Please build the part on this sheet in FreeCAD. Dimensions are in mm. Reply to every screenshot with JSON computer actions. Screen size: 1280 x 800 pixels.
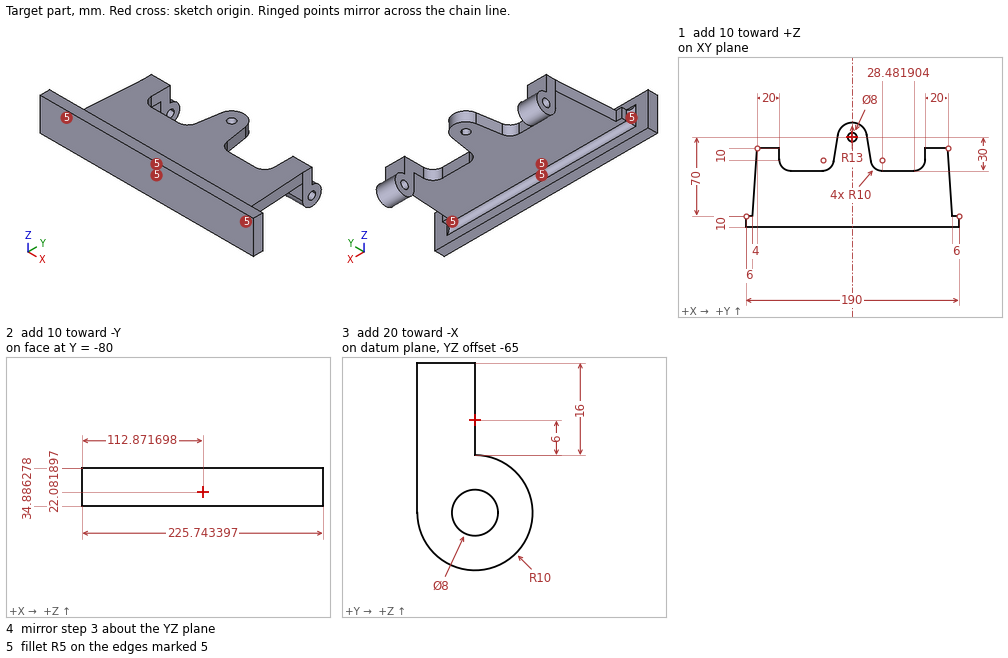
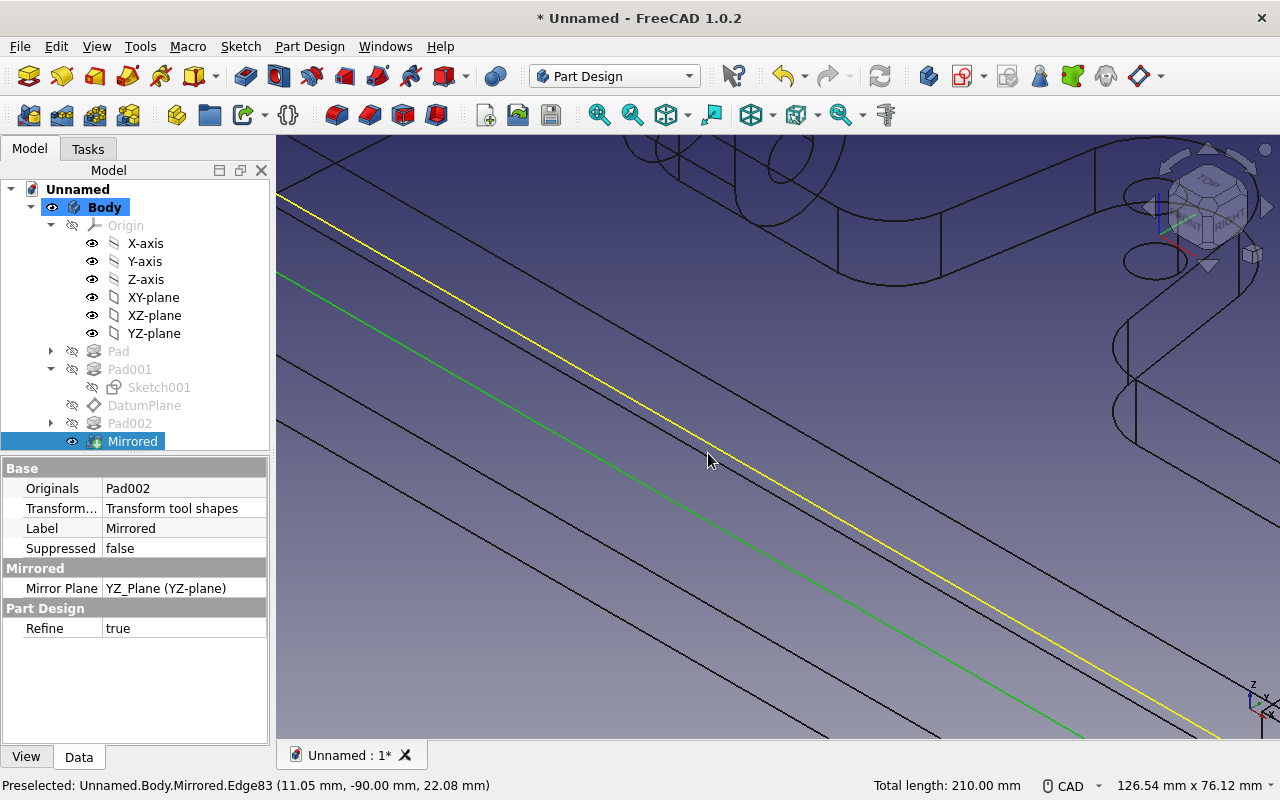
{"action": "left_click", "coordinate": [707, 455], "text": "ctrl"}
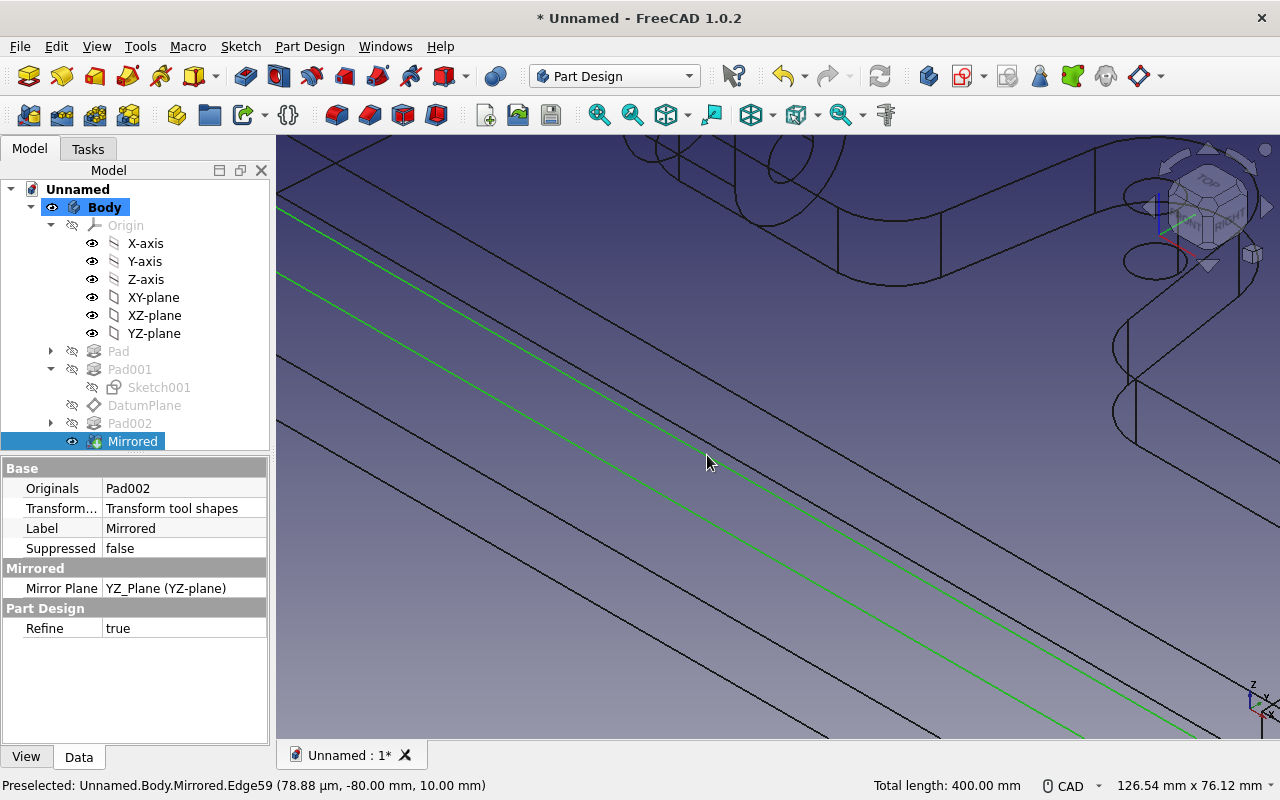
{"action": "key", "text": "v 1"}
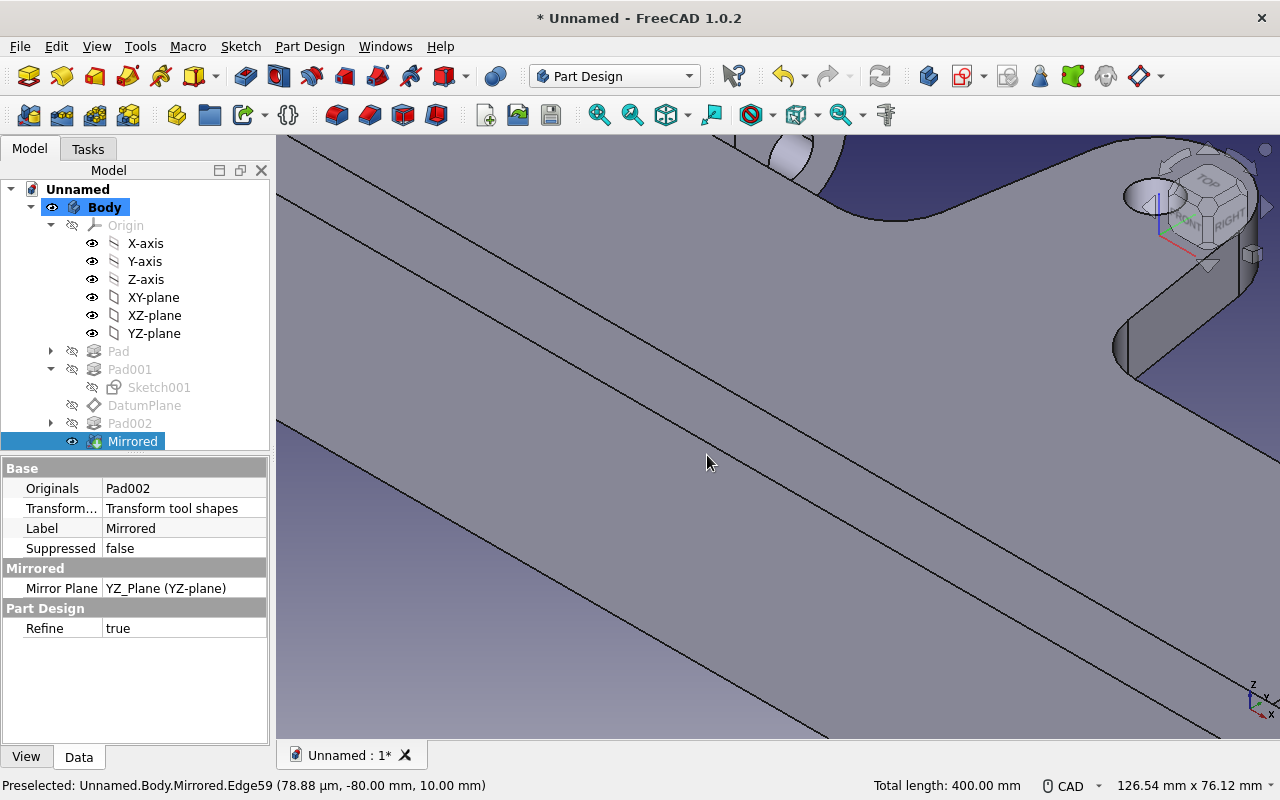
{"action": "left_click", "coordinate": [337, 116]}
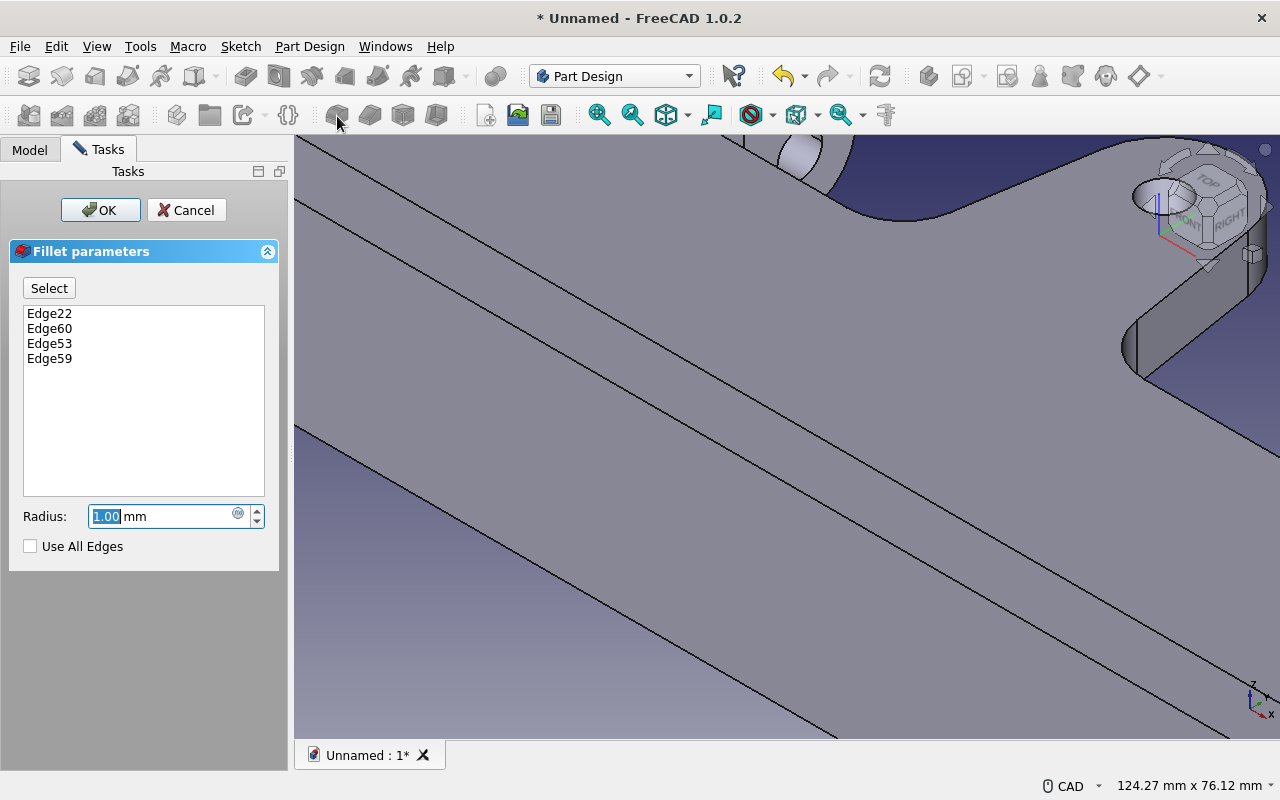
{"action": "type", "text": "5"}
{"action": "key", "text": "Tab"}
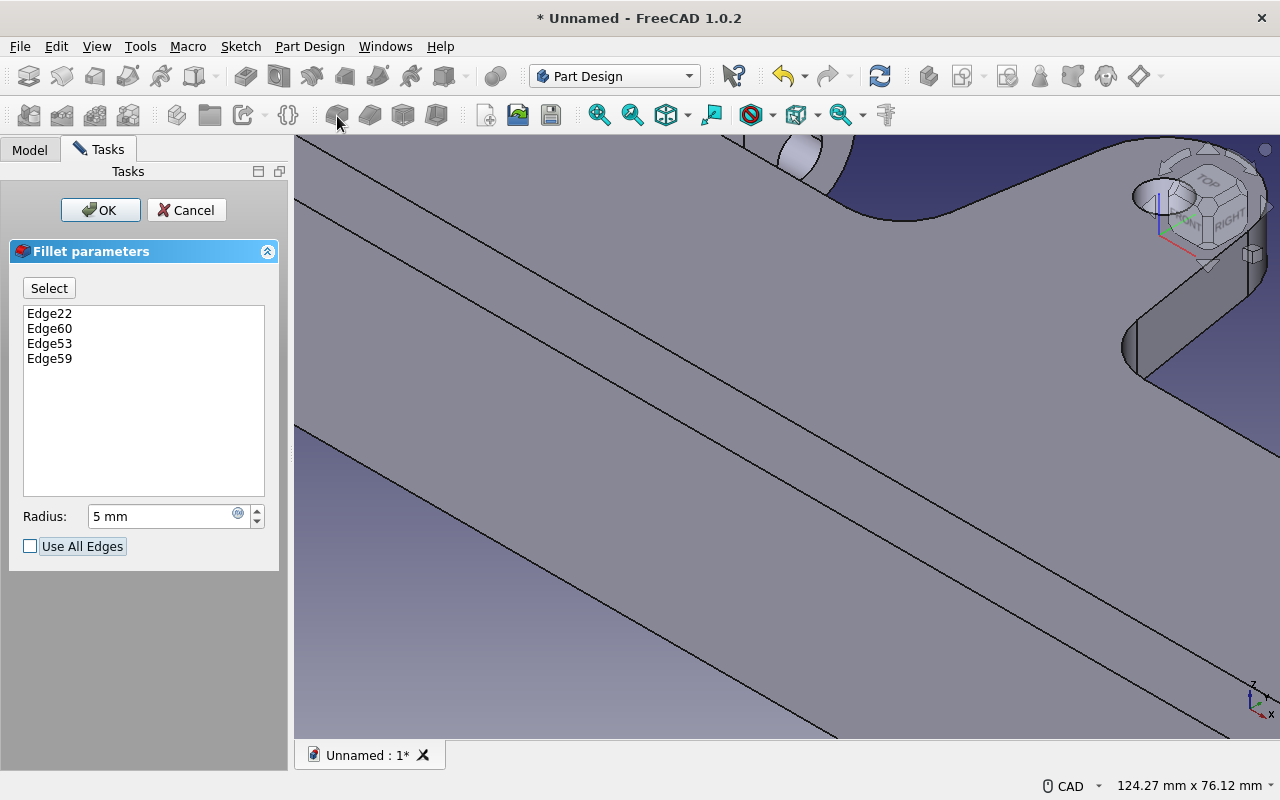
{"action": "left_click", "coordinate": [101, 210]}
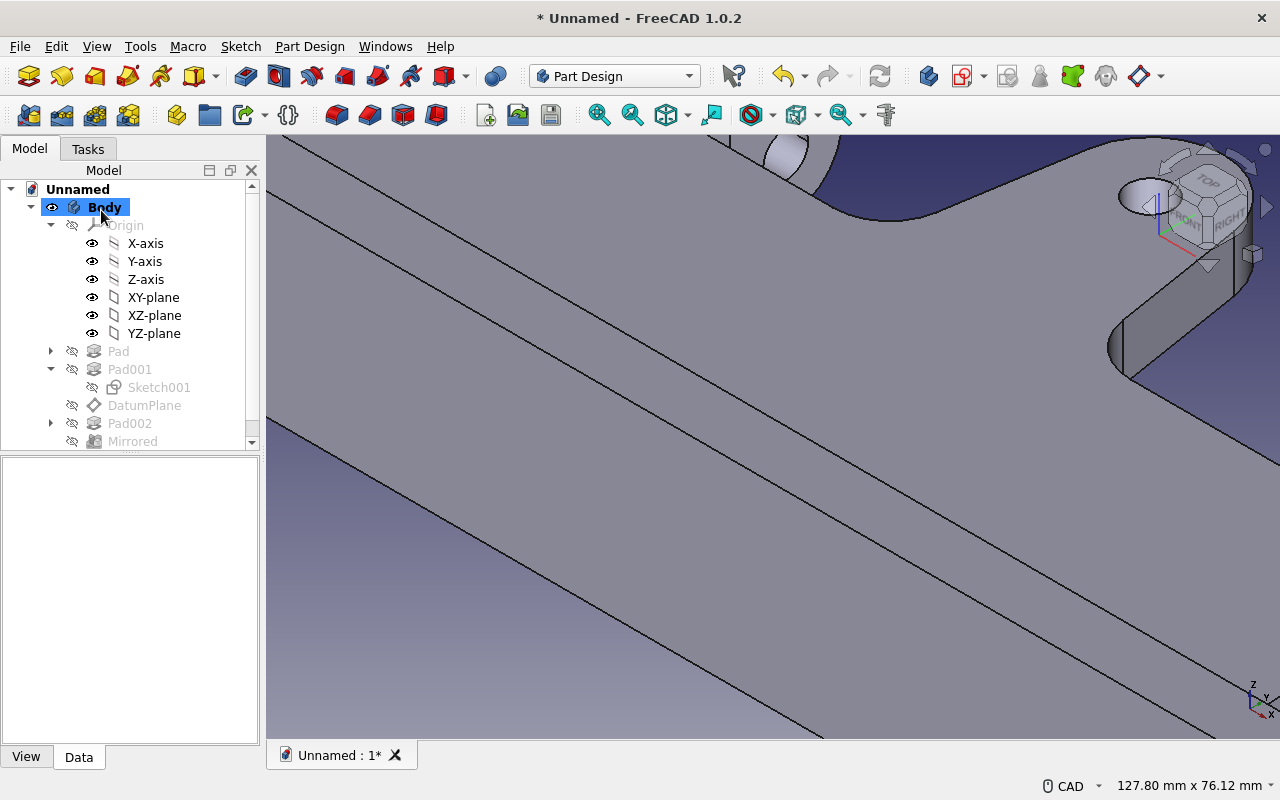
{"action": "left_click", "coordinate": [600, 116]}